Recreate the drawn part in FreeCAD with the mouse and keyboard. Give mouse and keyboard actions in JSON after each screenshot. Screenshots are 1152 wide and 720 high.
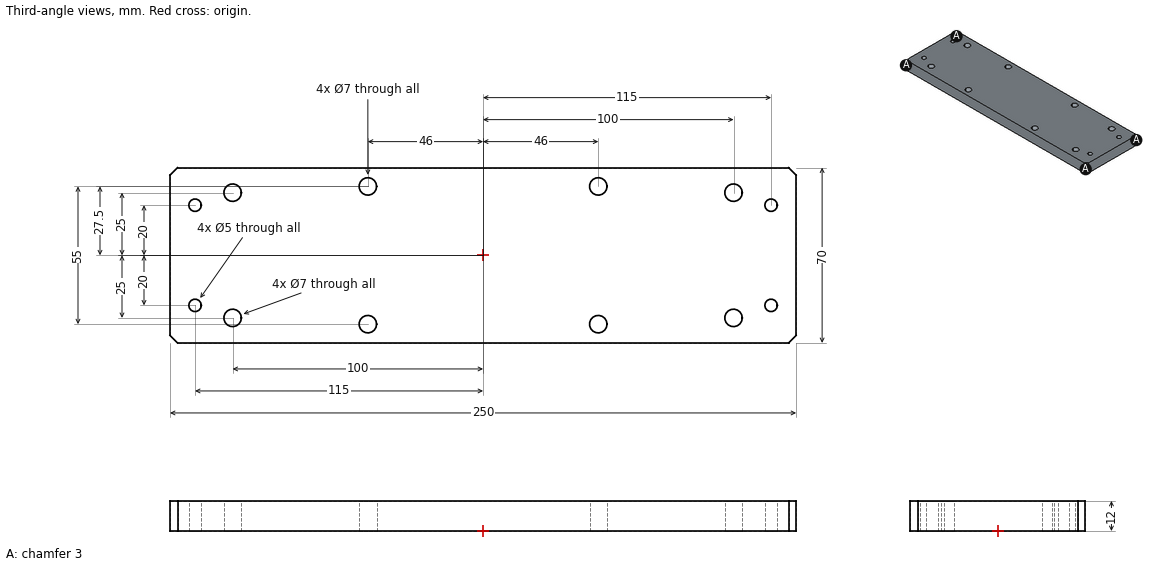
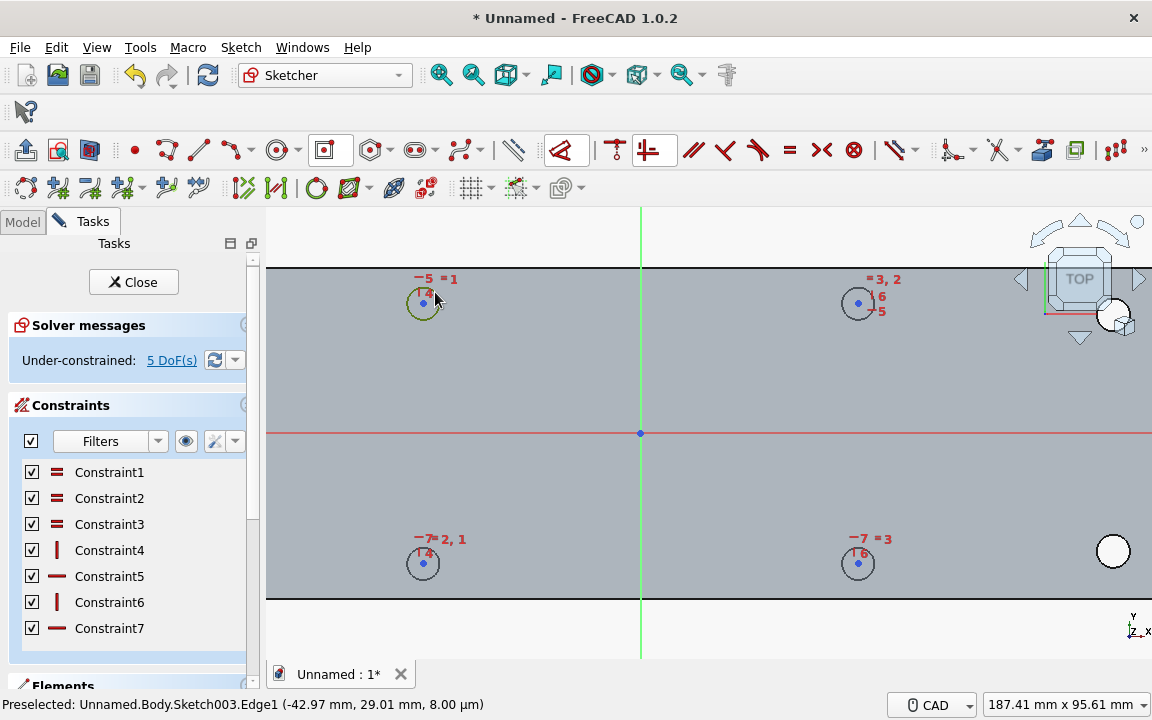
{"action": "left_click", "coordinate": [584, 150]}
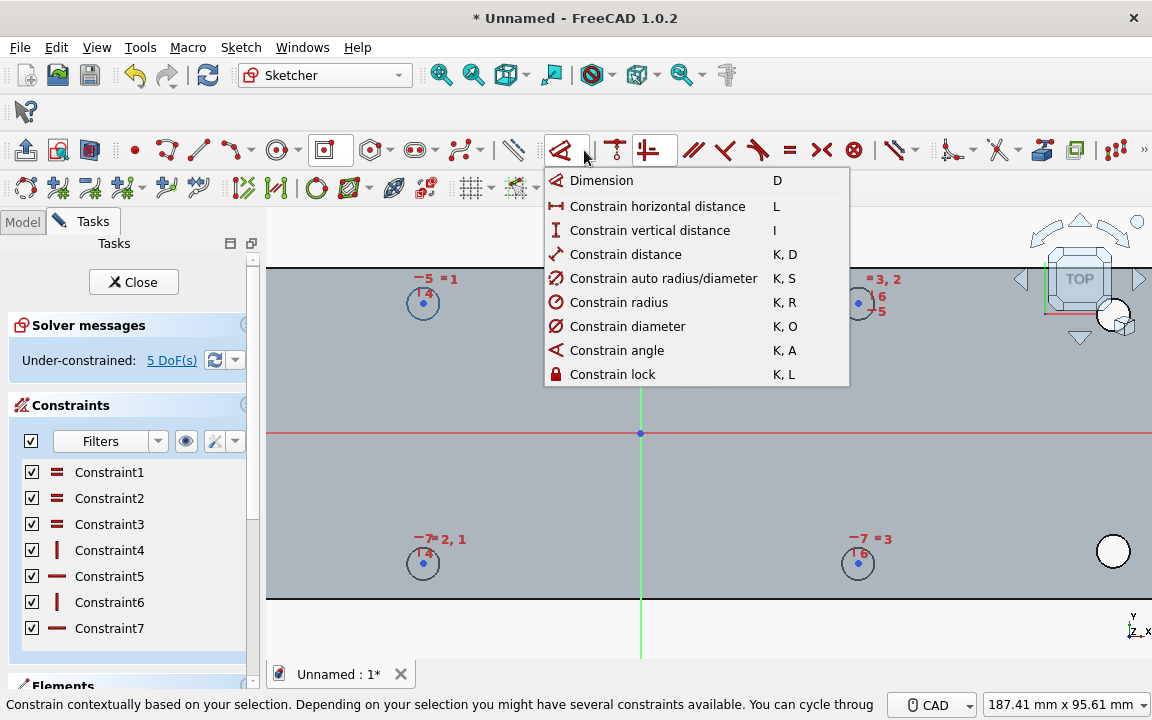
{"action": "left_click", "coordinate": [697, 326]}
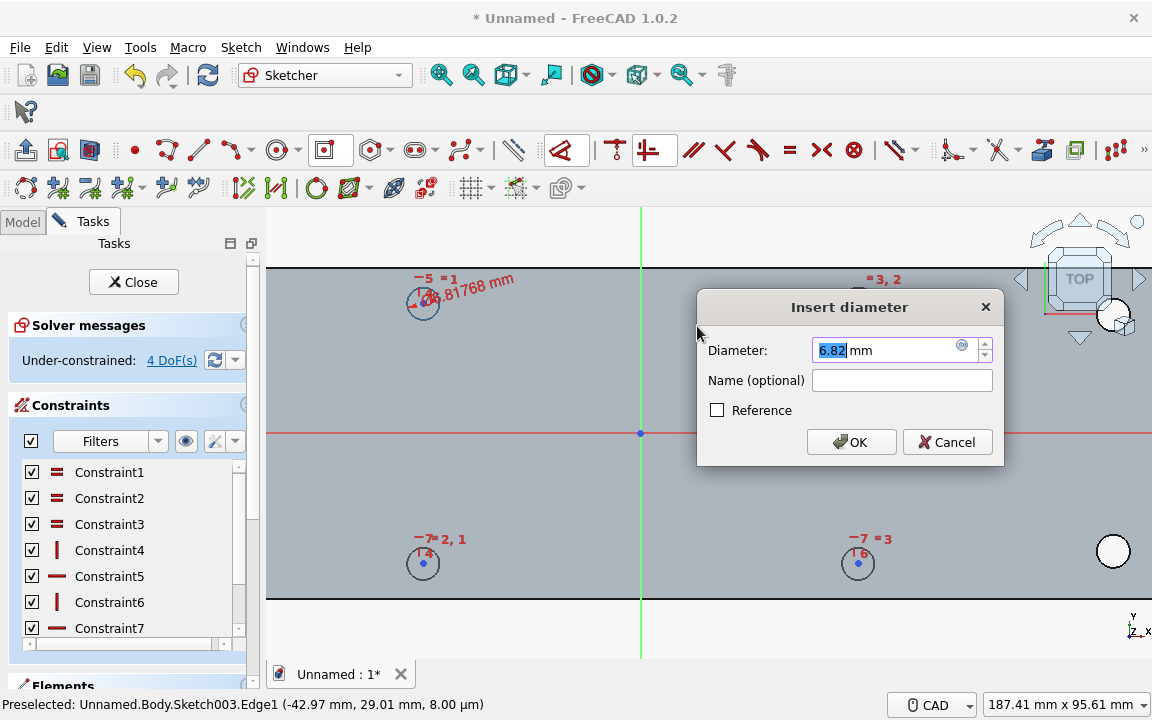
{"action": "type", "text": "7"}
{"action": "key", "text": "Return"}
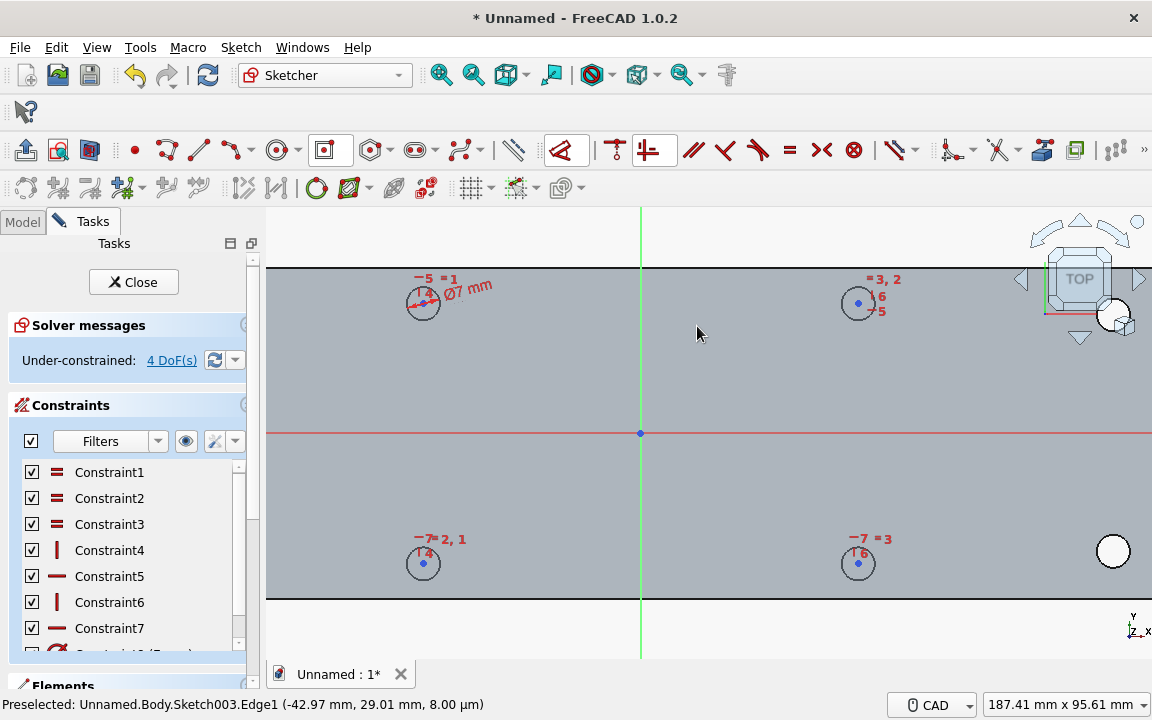
{"action": "left_click", "coordinate": [423, 304]}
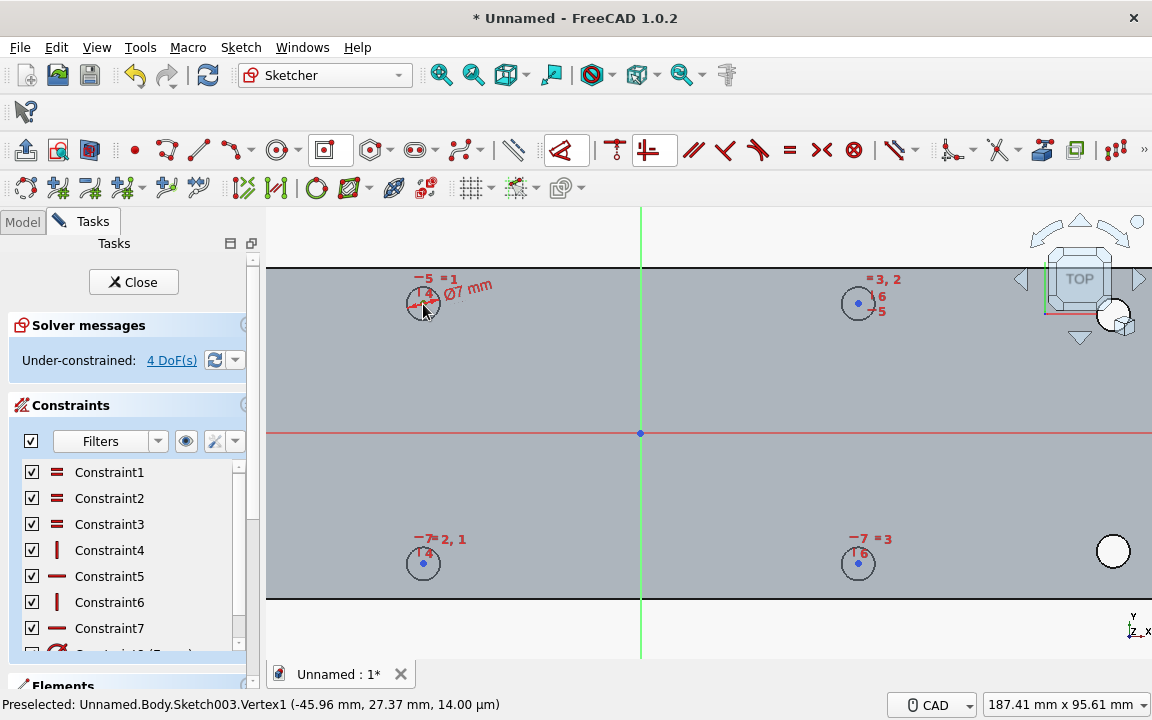
{"action": "left_click", "coordinate": [584, 150]}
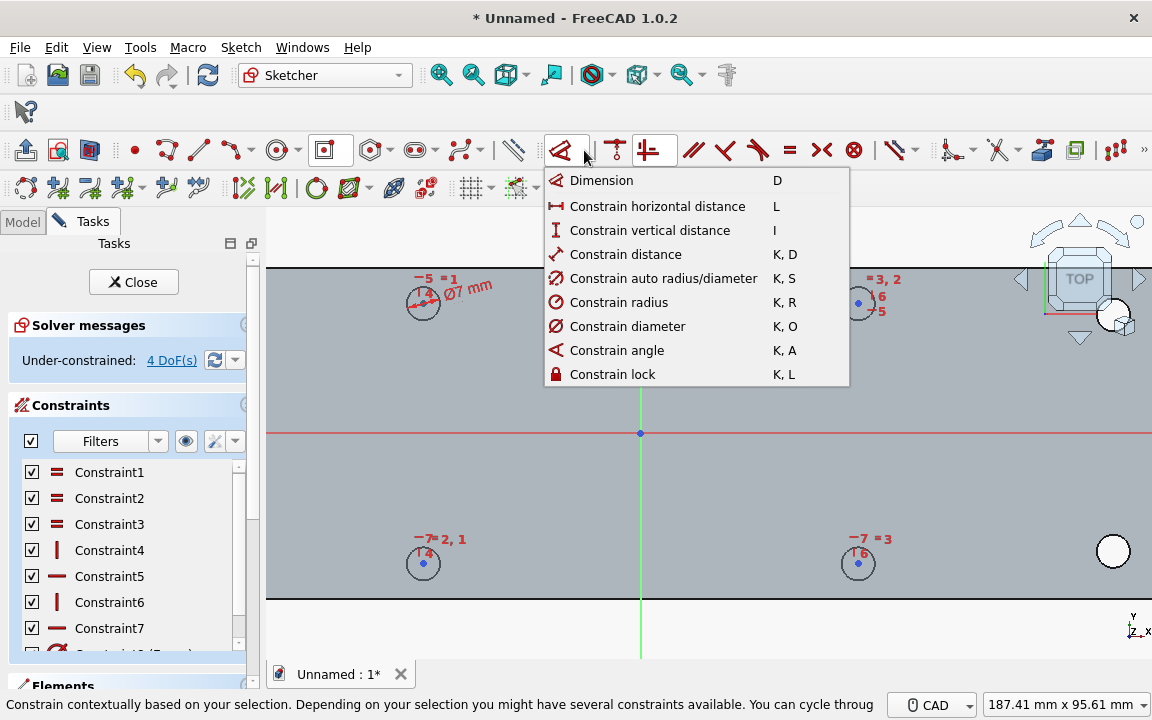
{"action": "left_click", "coordinate": [697, 206]}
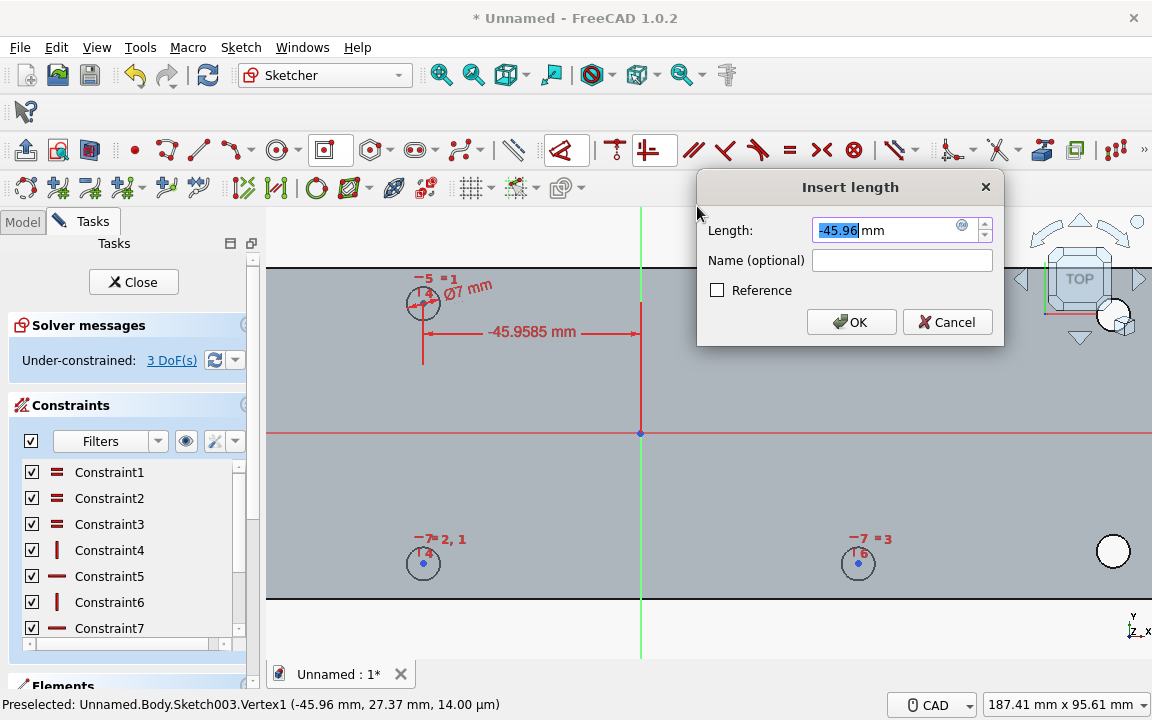
{"action": "type", "text": "-46"}
{"action": "key", "text": "Return"}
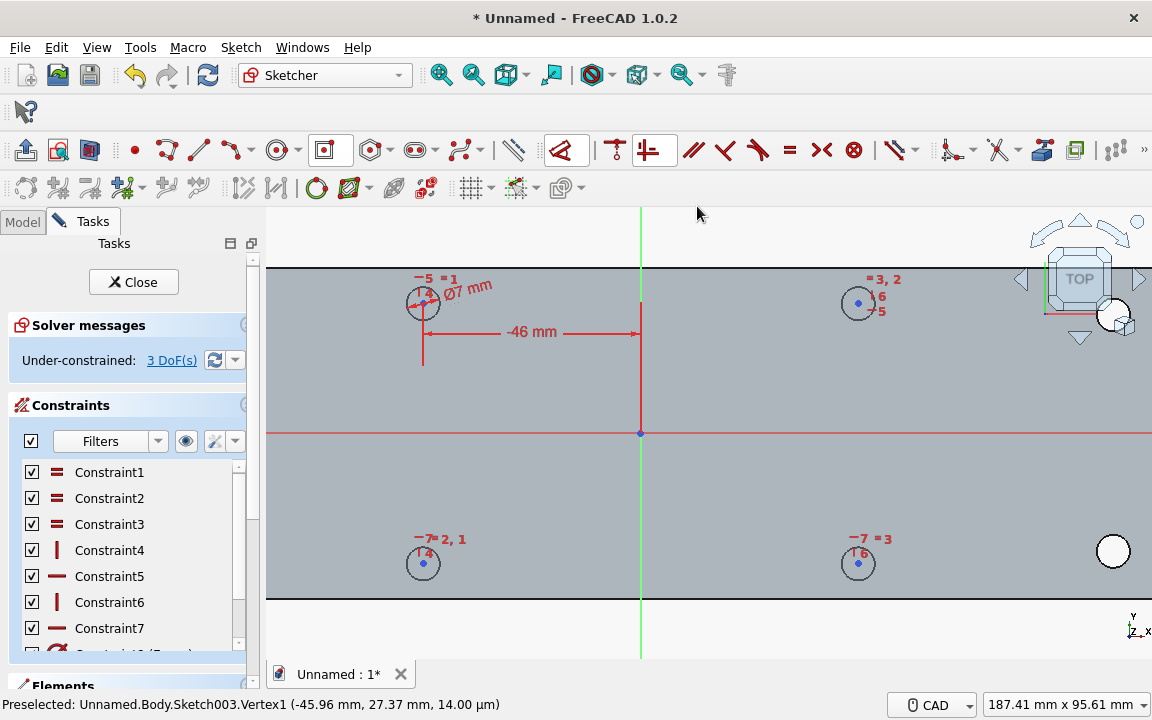
{"action": "left_click", "coordinate": [858, 304]}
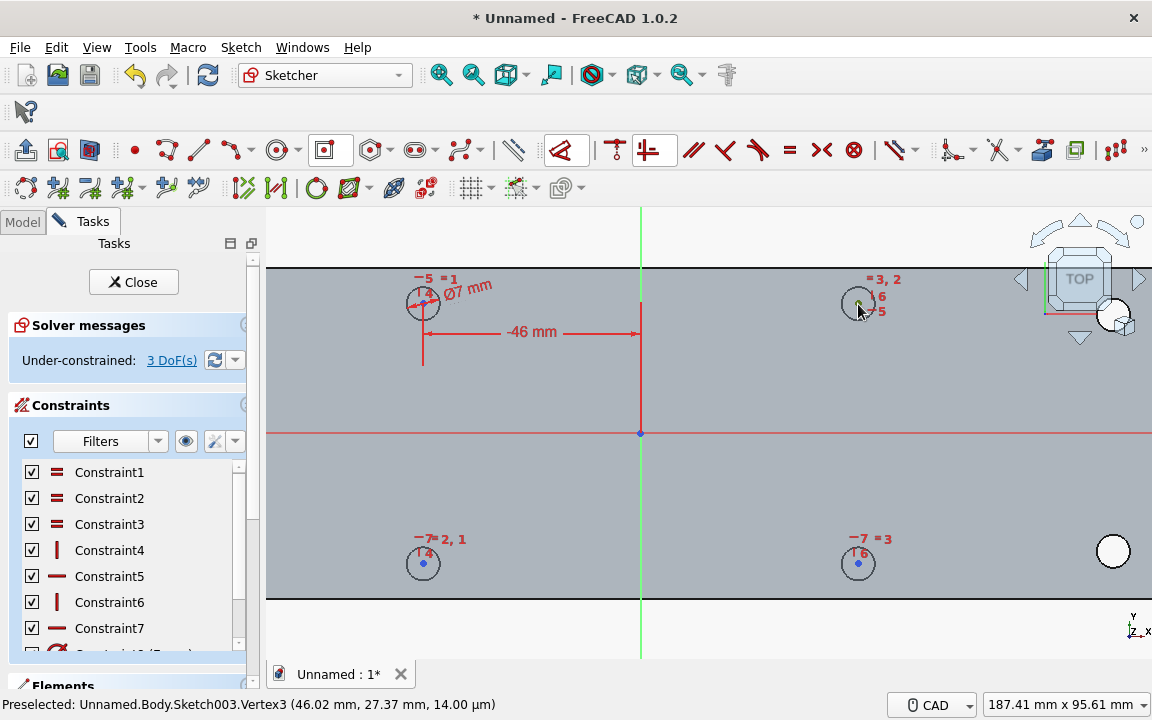
{"action": "key", "text": "l"}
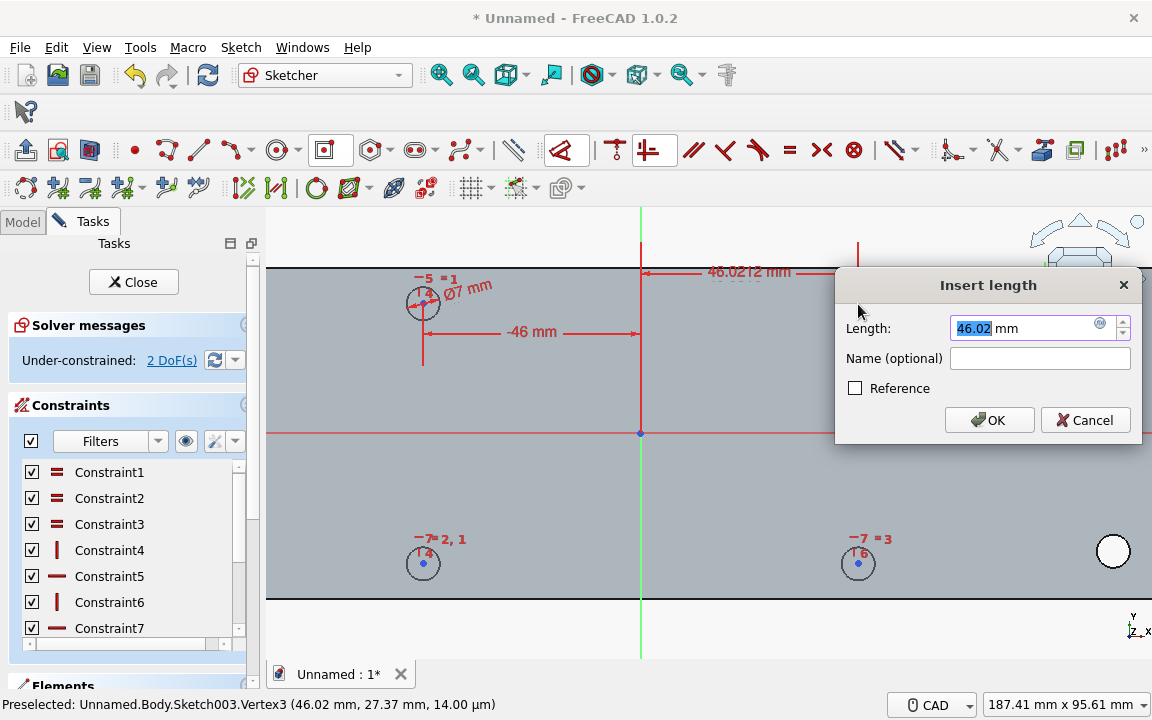
{"action": "type", "text": "46"}
{"action": "key", "text": "Return"}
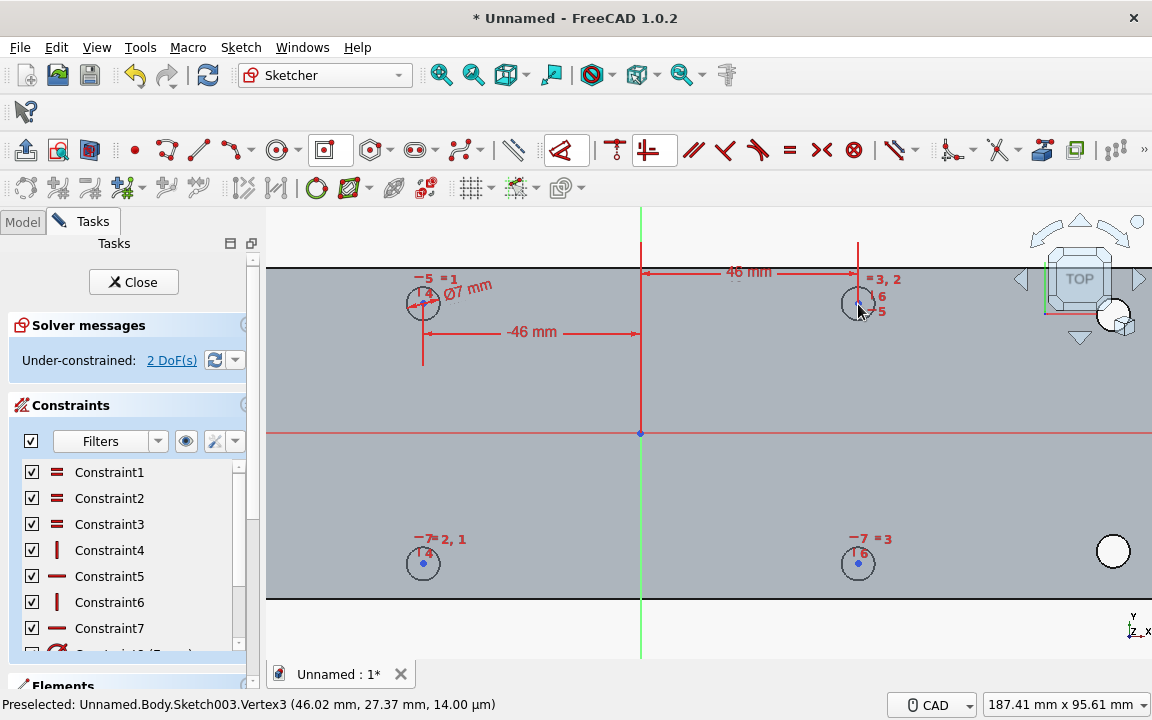
{"action": "left_click", "coordinate": [423, 304]}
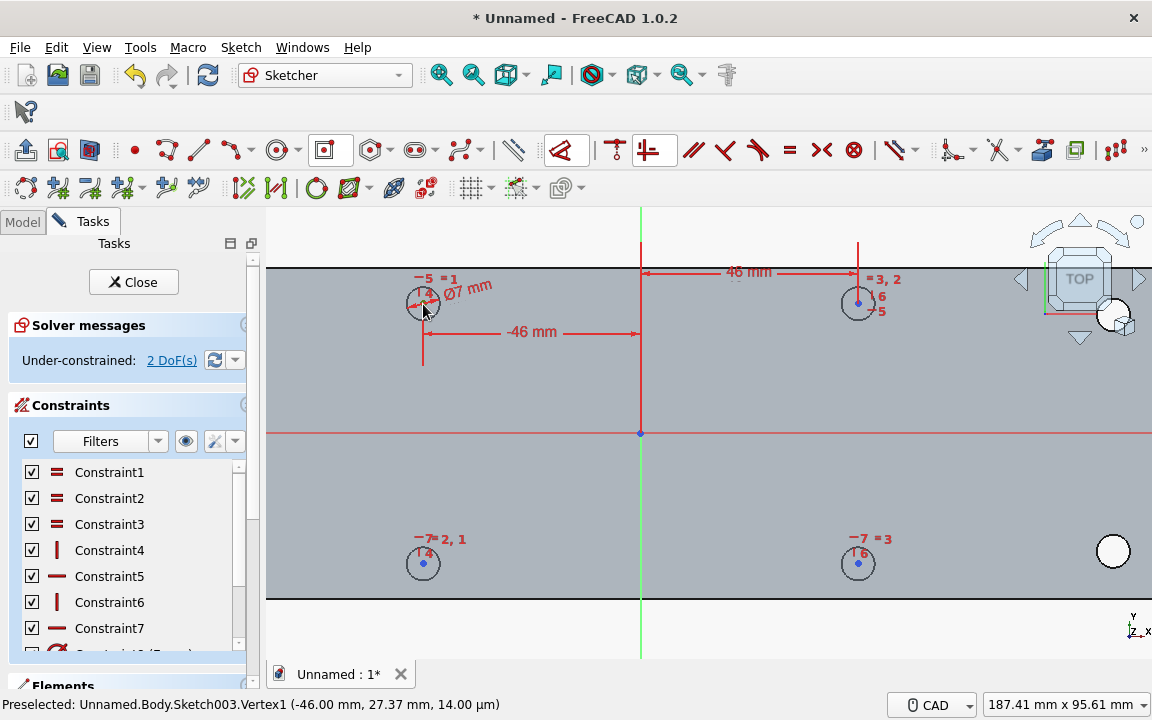
{"action": "left_click", "coordinate": [423, 564]}